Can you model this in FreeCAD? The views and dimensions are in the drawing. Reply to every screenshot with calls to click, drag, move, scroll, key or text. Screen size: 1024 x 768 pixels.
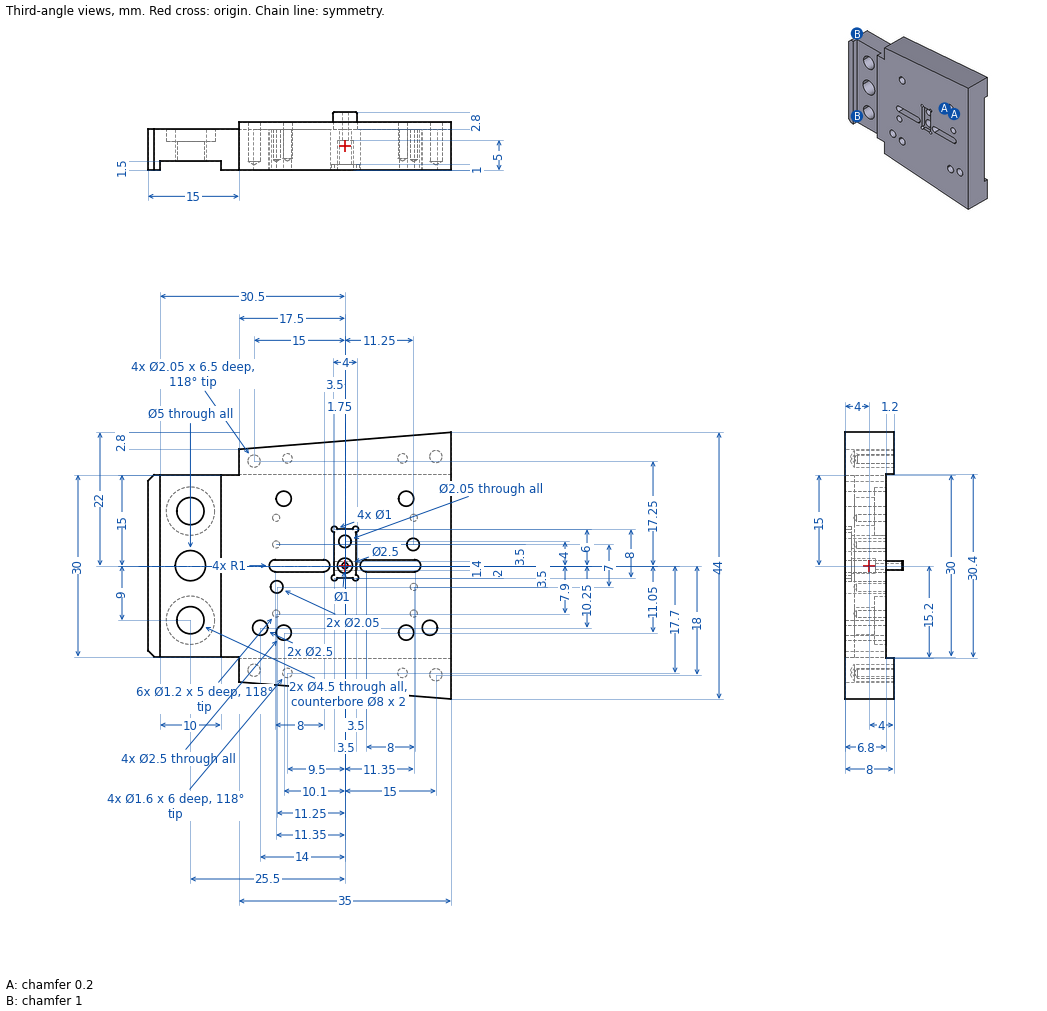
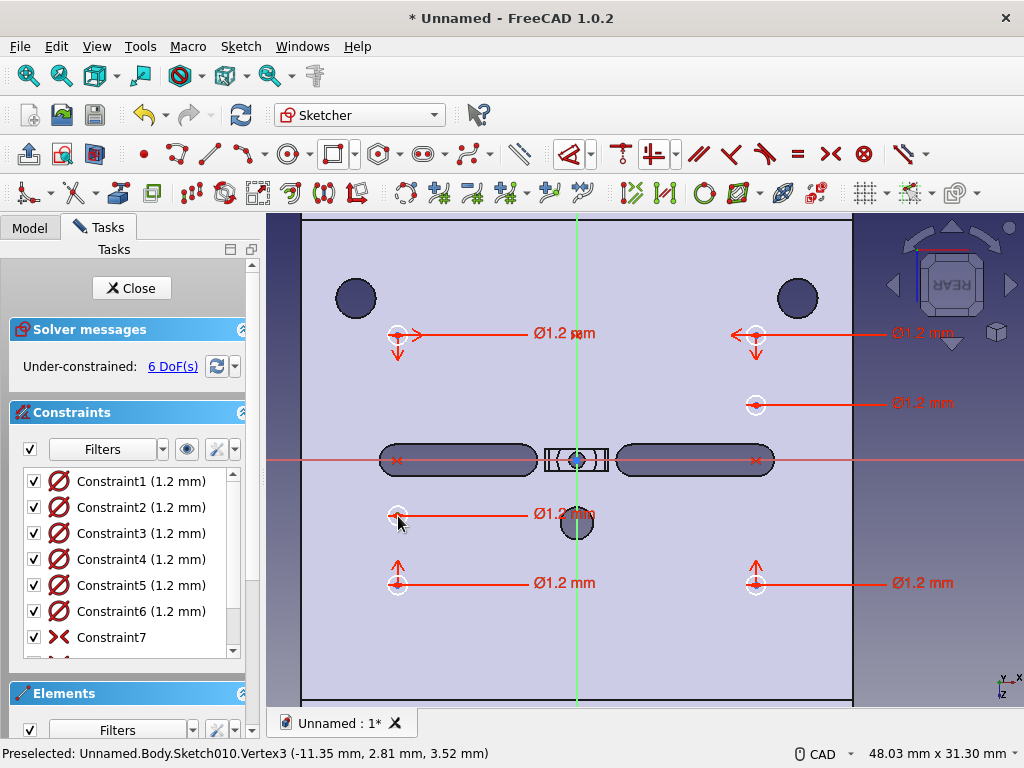
click(756, 405)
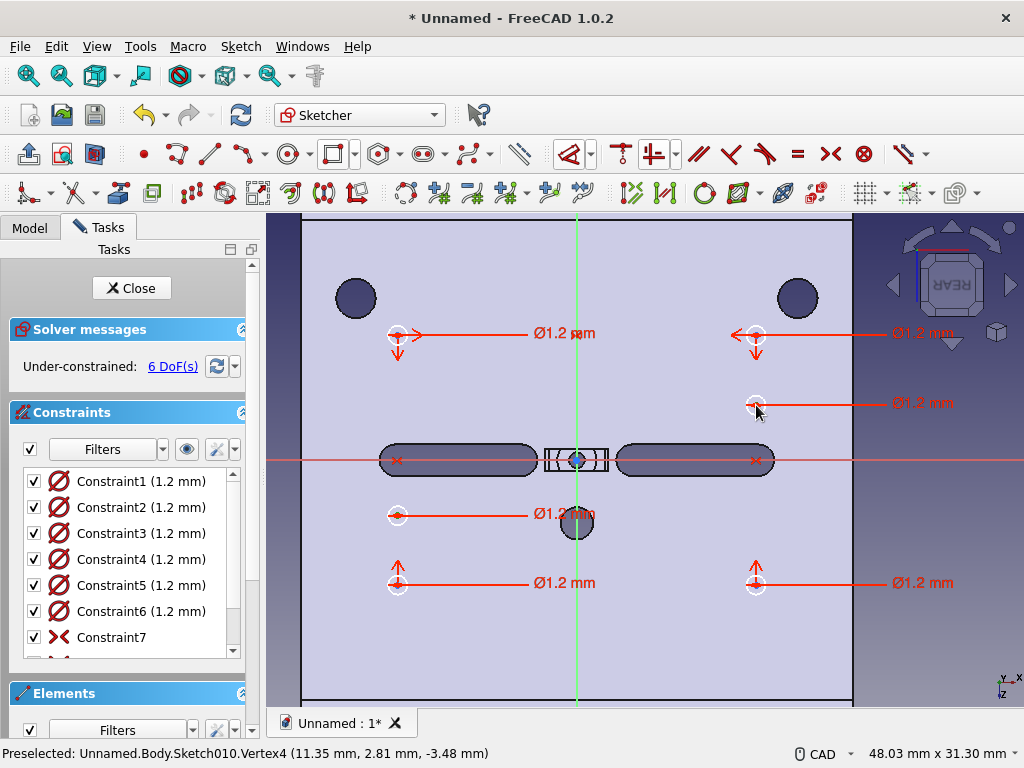
click(590, 154)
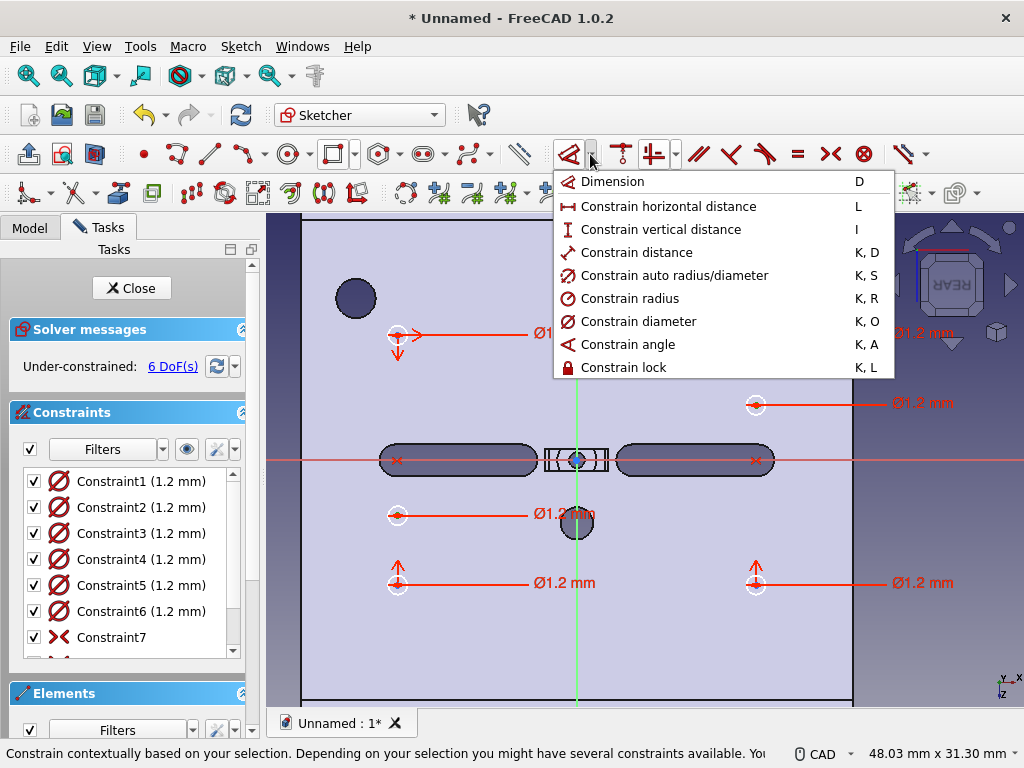
click(724, 230)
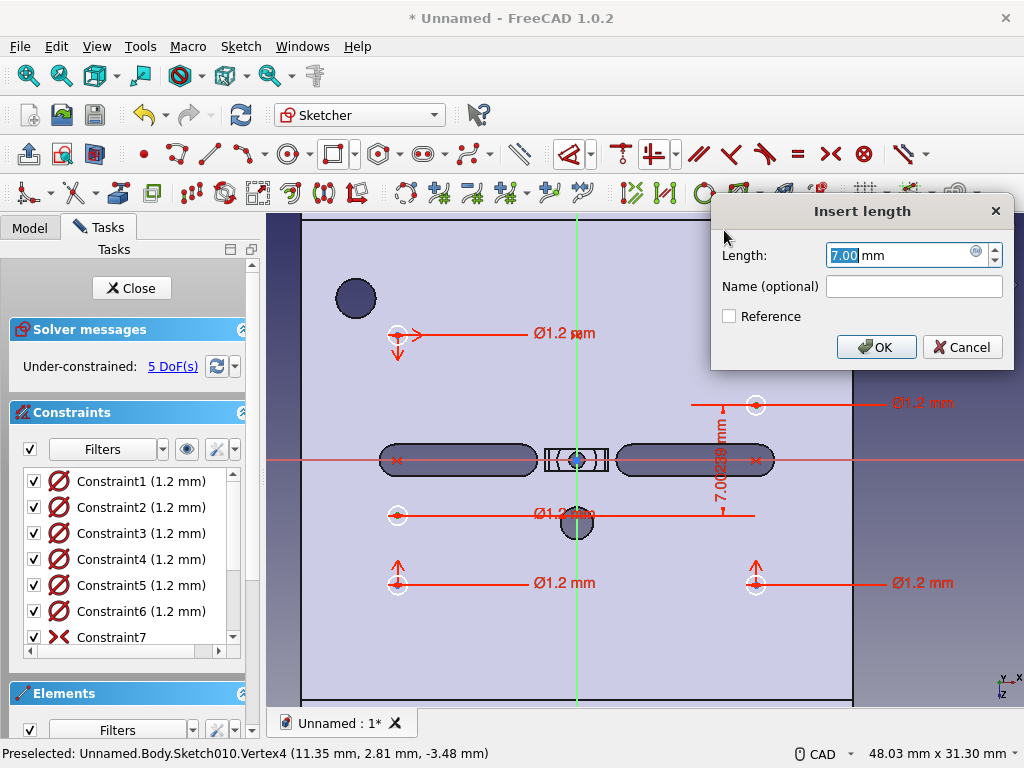
text(7)
key(Return)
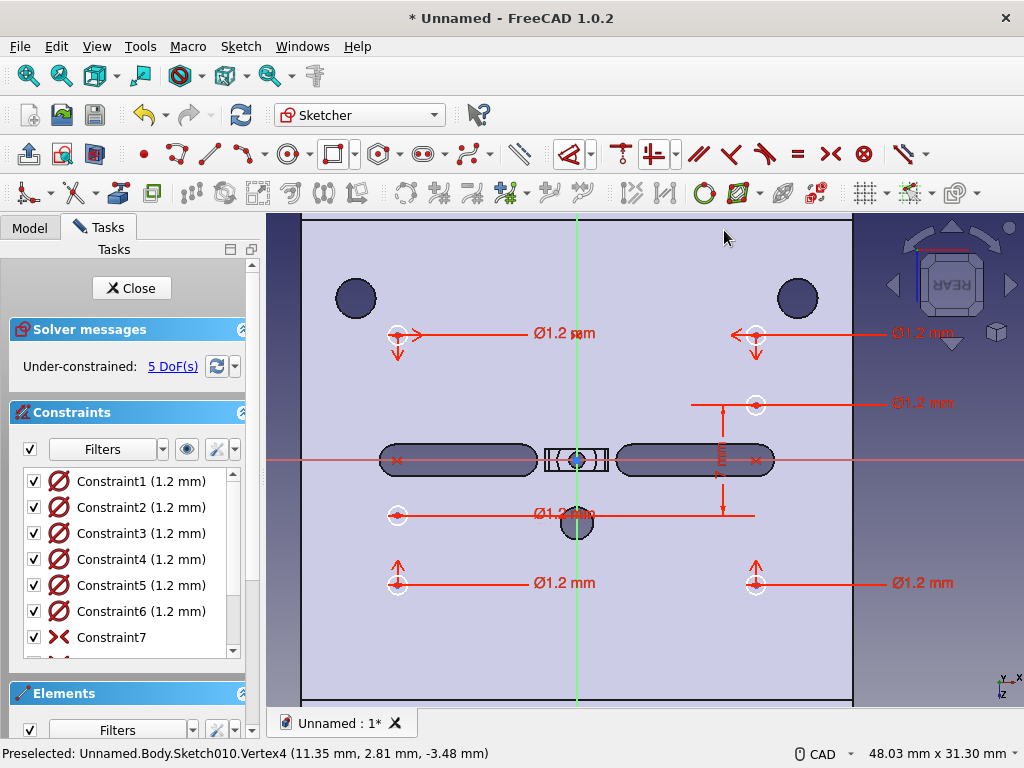
click(398, 335)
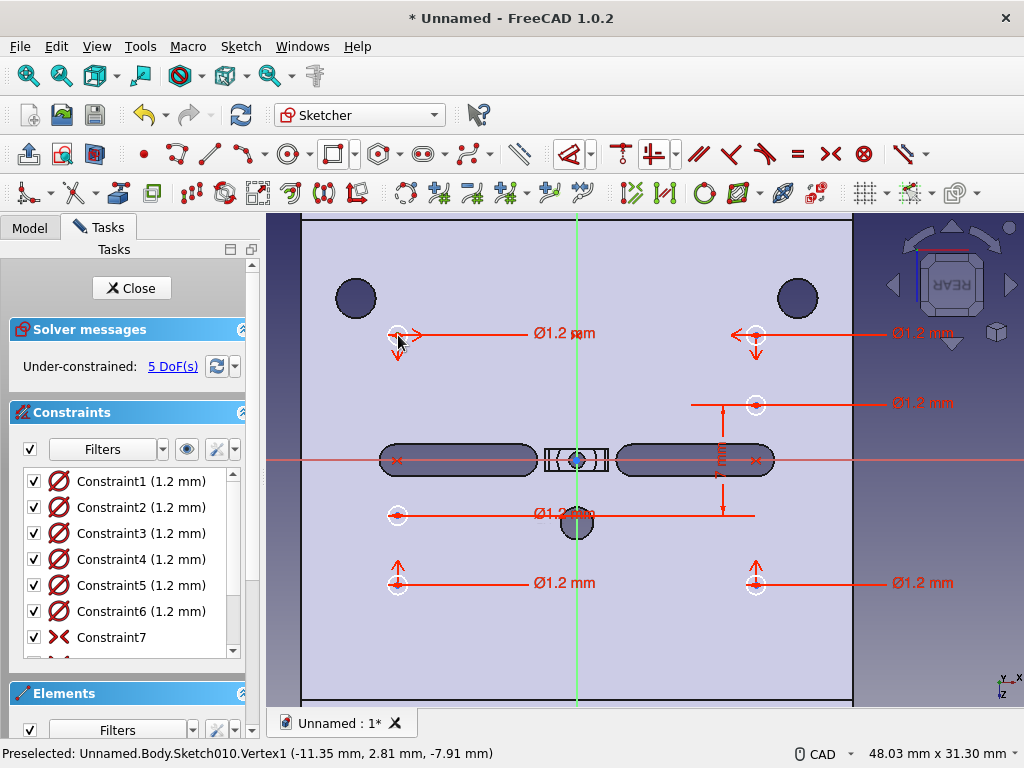
click(590, 154)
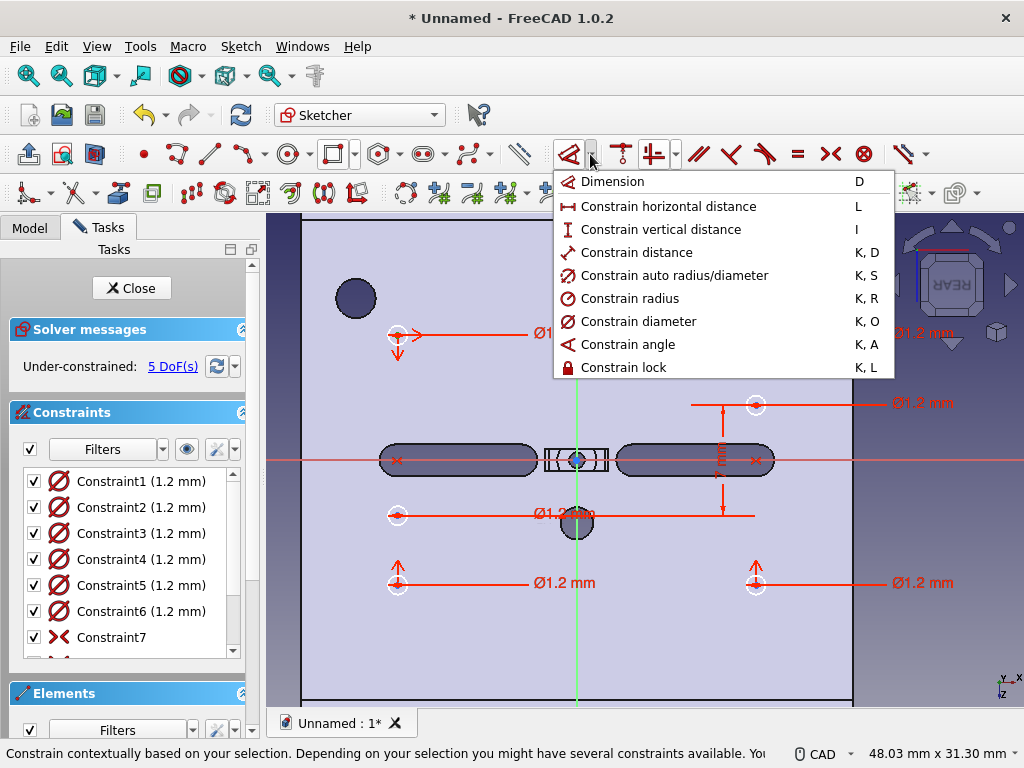
click(724, 230)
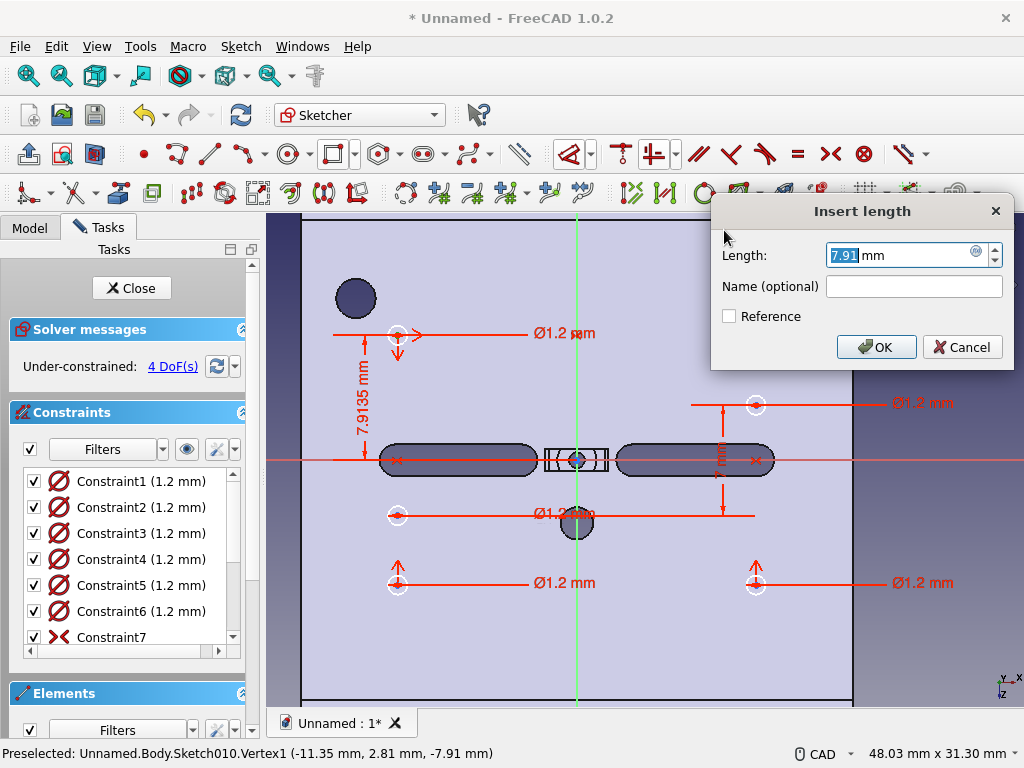
text(7.9)
key(Return)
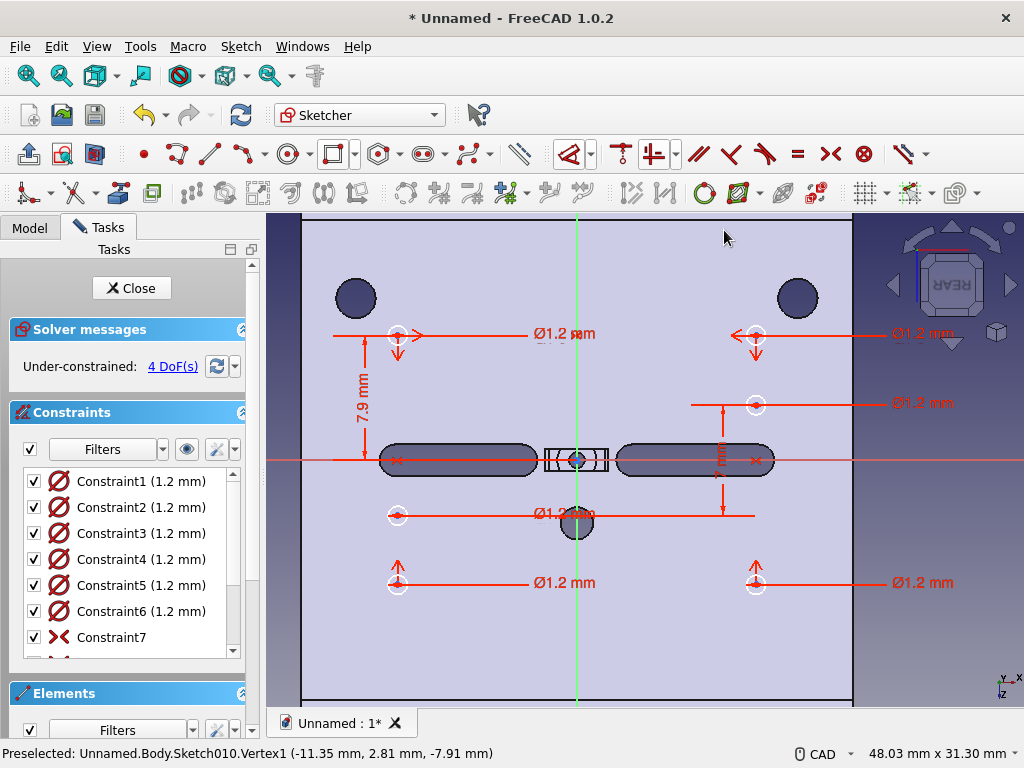
click(398, 516)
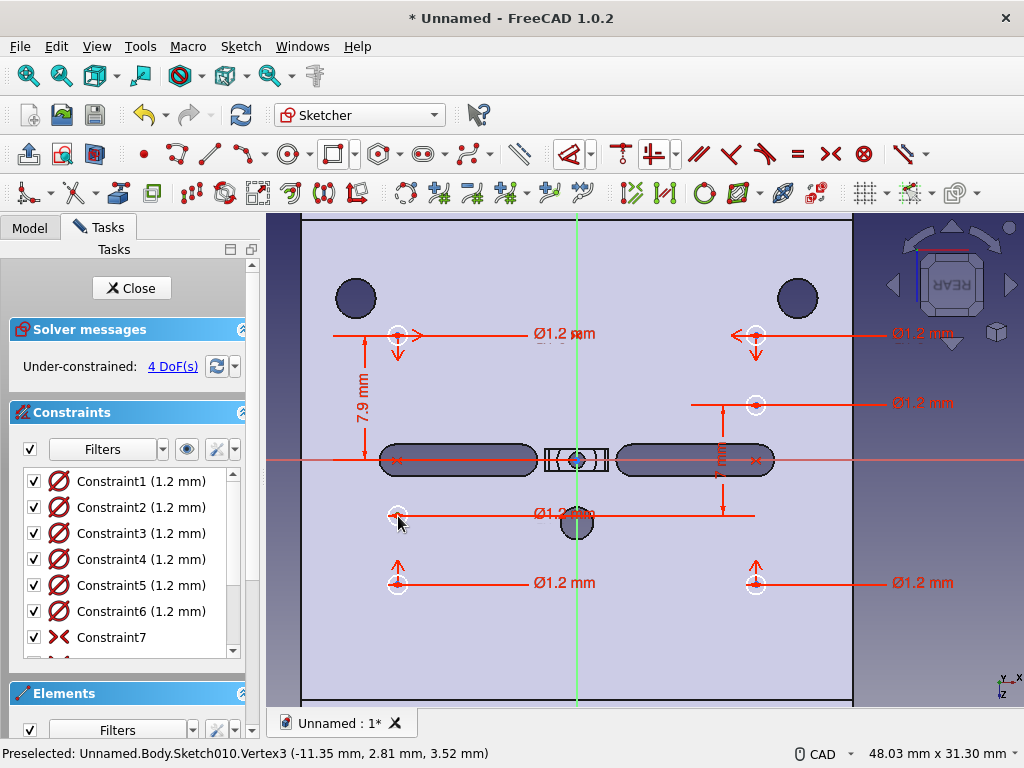
key(i)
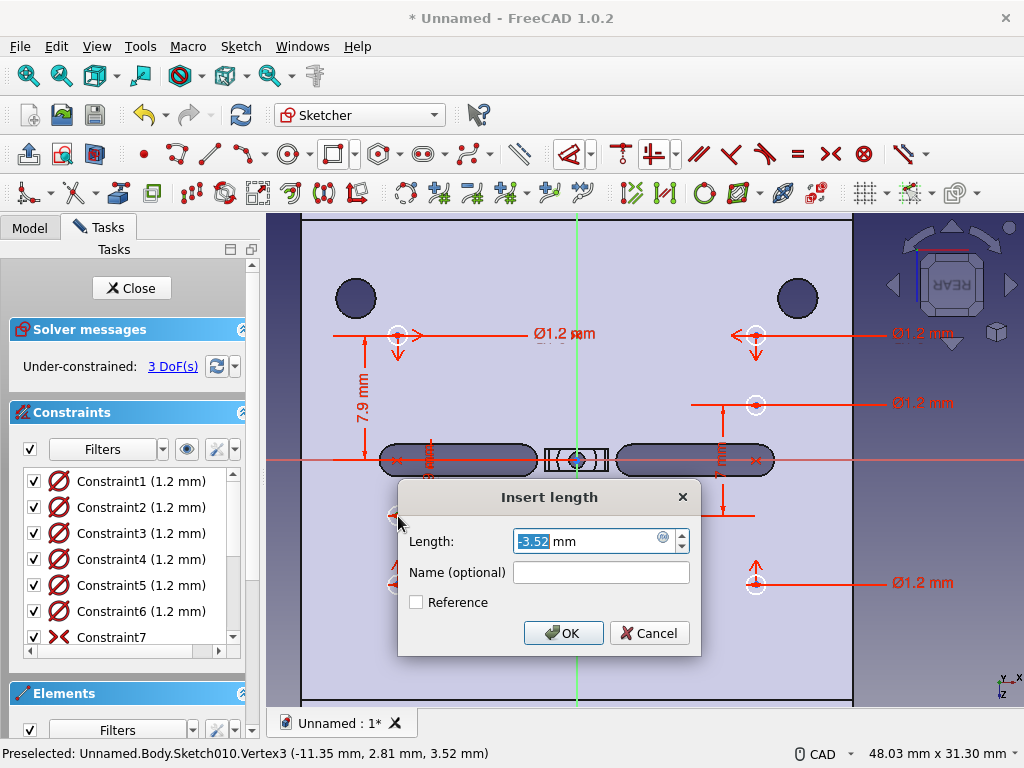
text(-3.5)
key(Return)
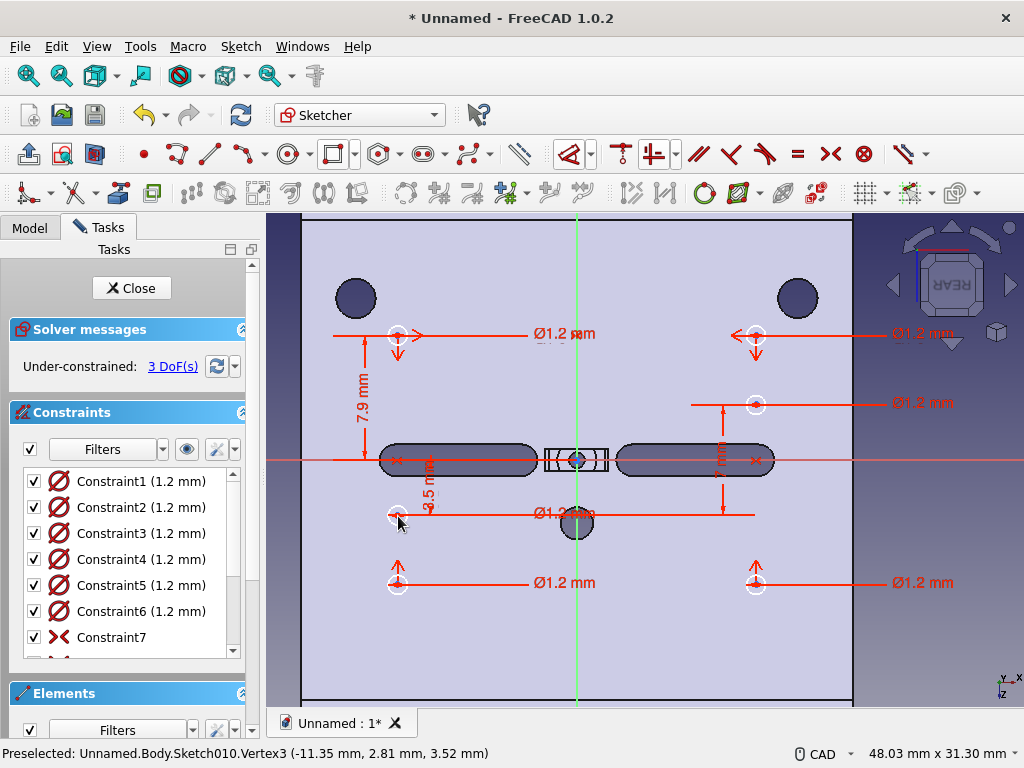
click(398, 336)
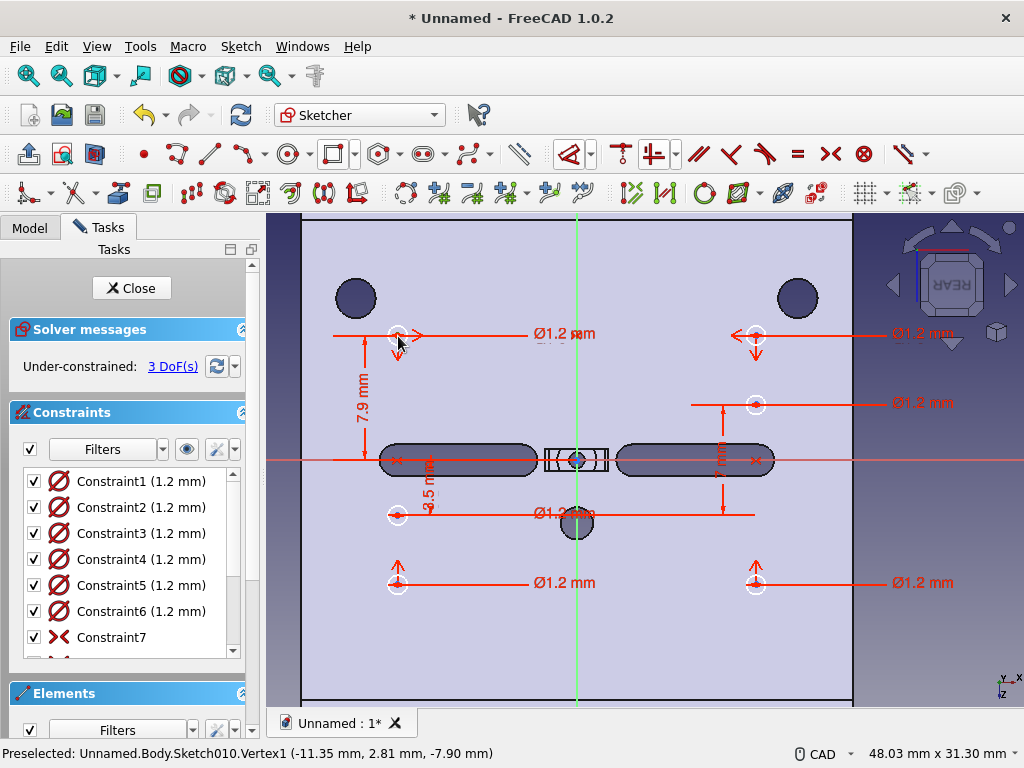
key(l)